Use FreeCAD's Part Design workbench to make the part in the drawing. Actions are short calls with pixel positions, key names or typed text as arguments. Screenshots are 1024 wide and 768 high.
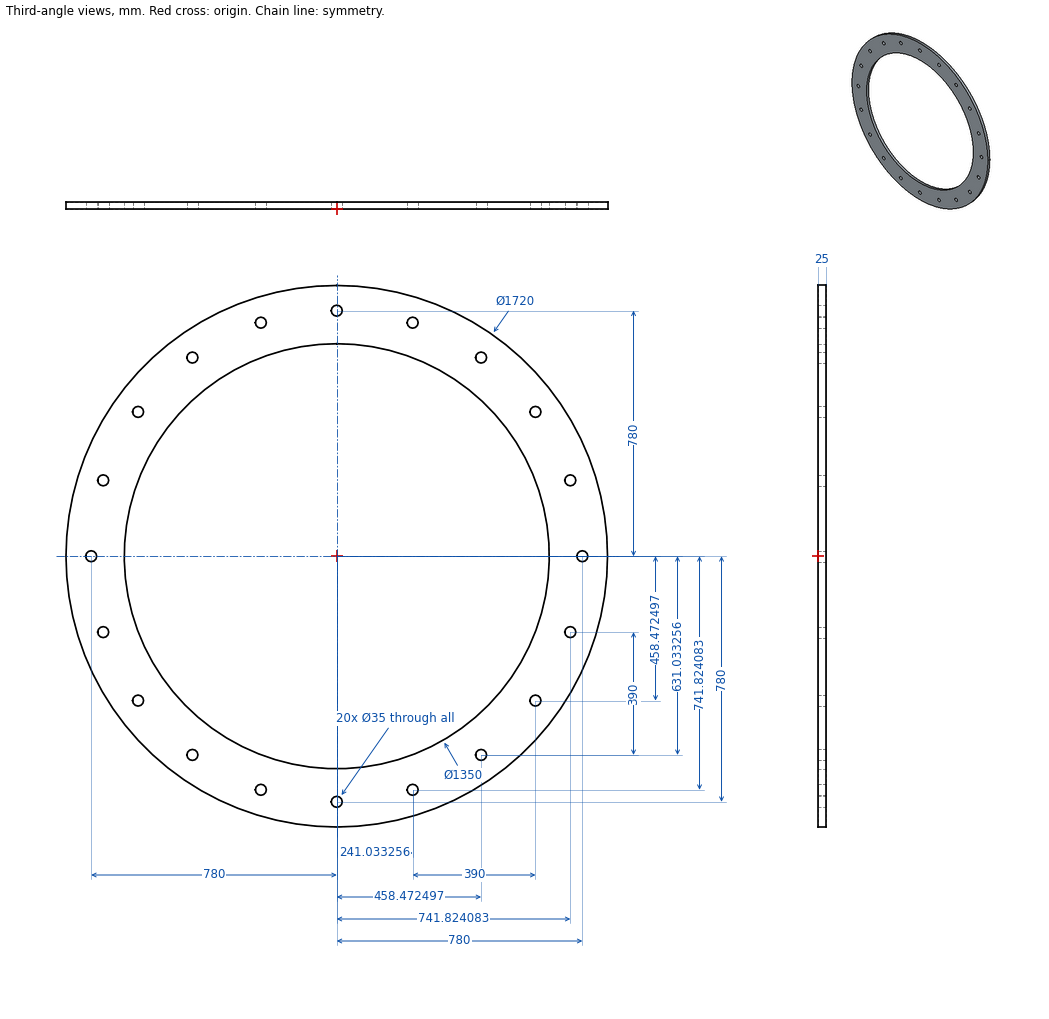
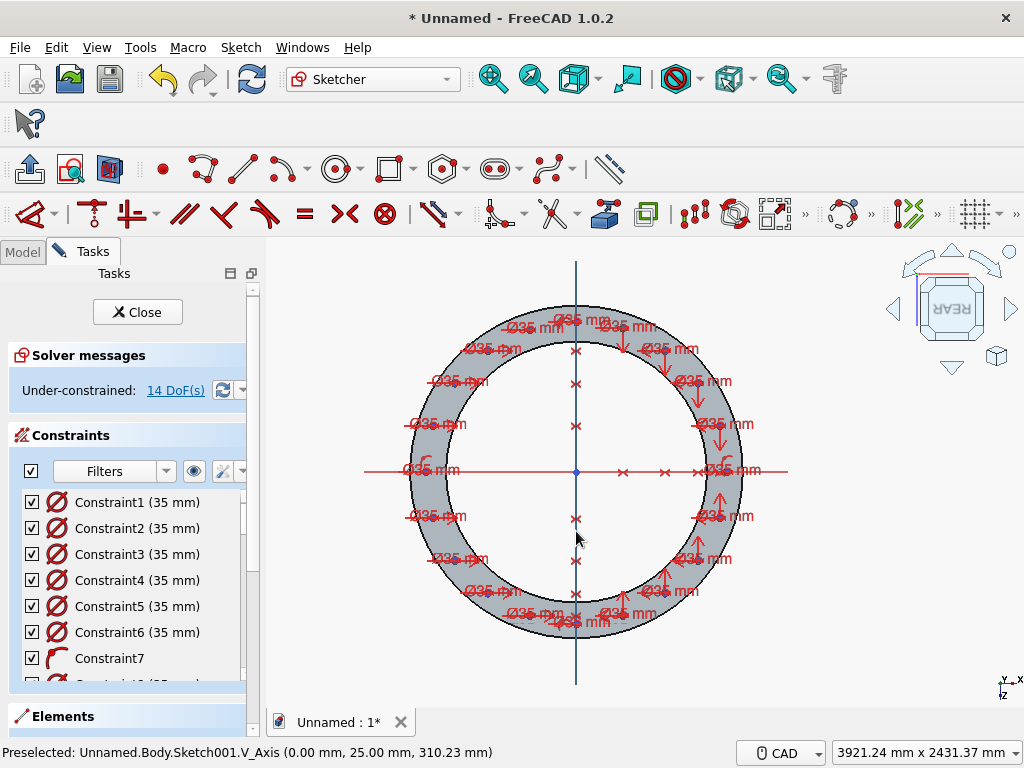
click(346, 214)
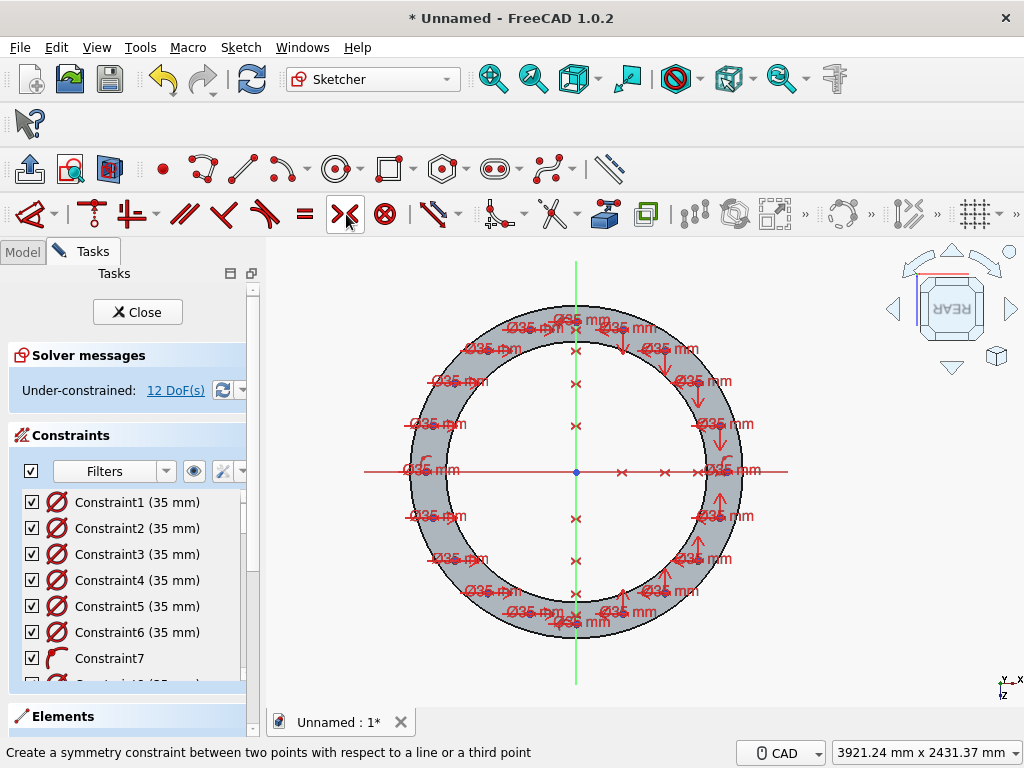
click(30, 214)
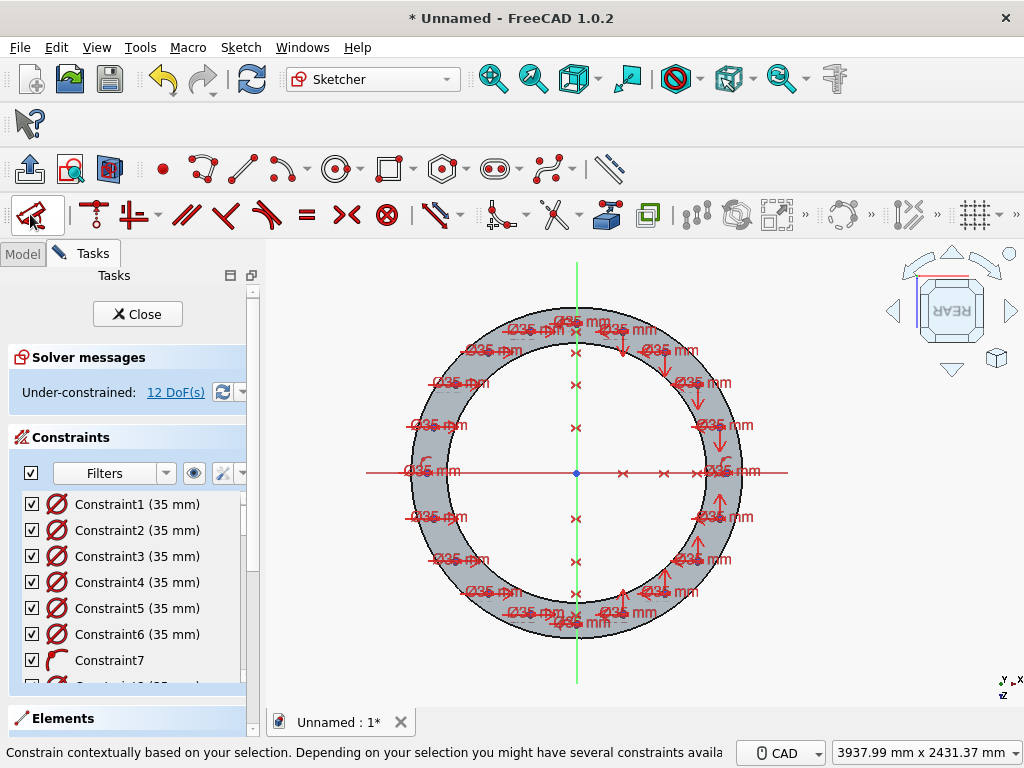
click(577, 324)
click(611, 398)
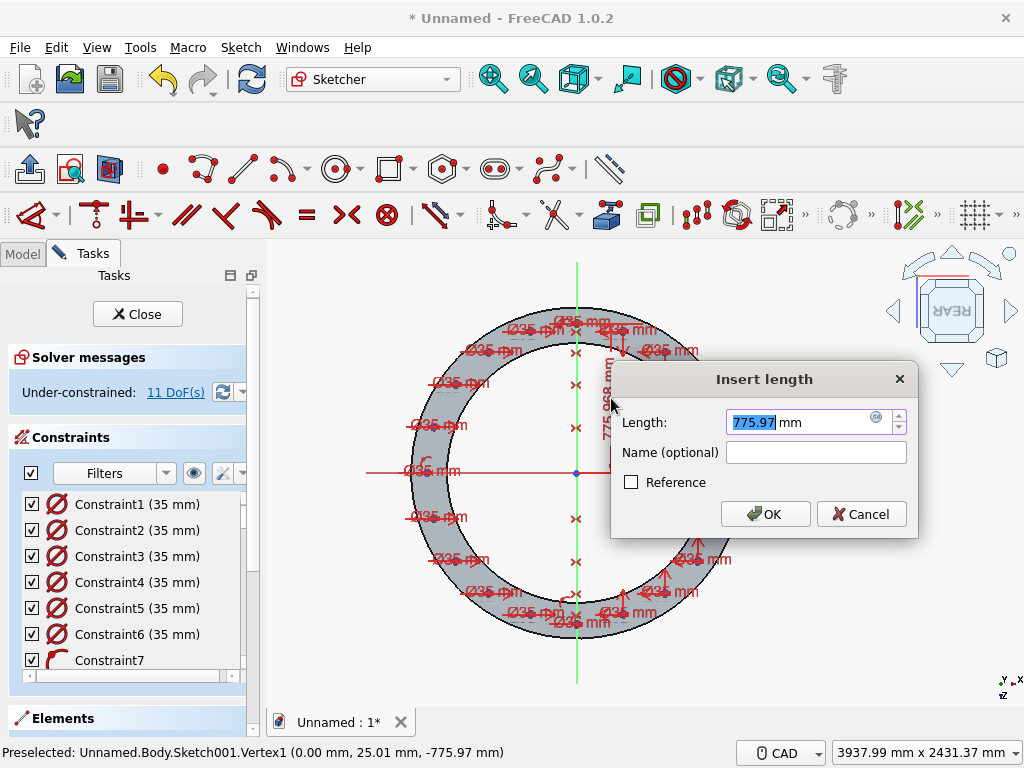
text(780)
key(Return)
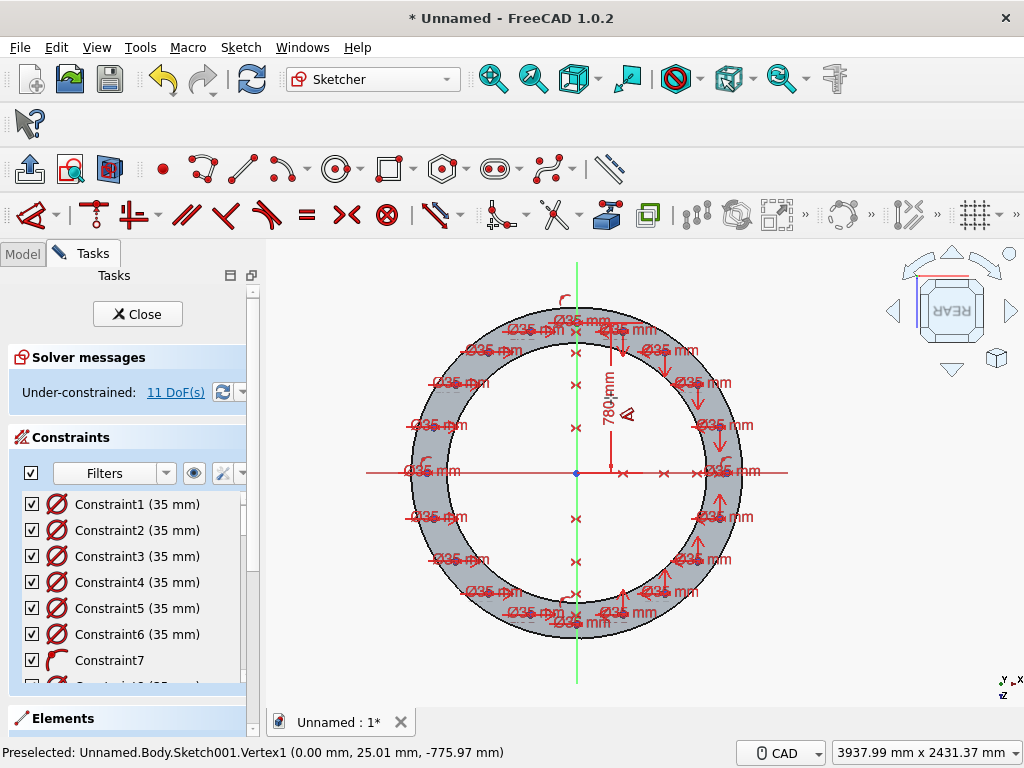
click(727, 473)
click(652, 507)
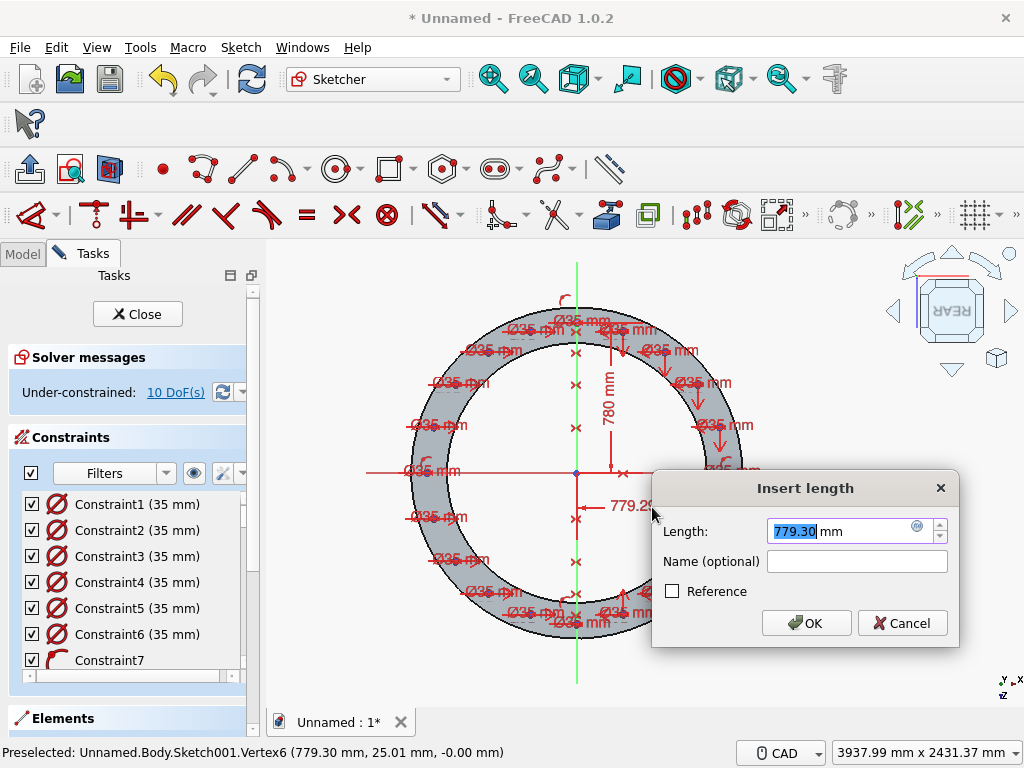
text(780)
key(Return)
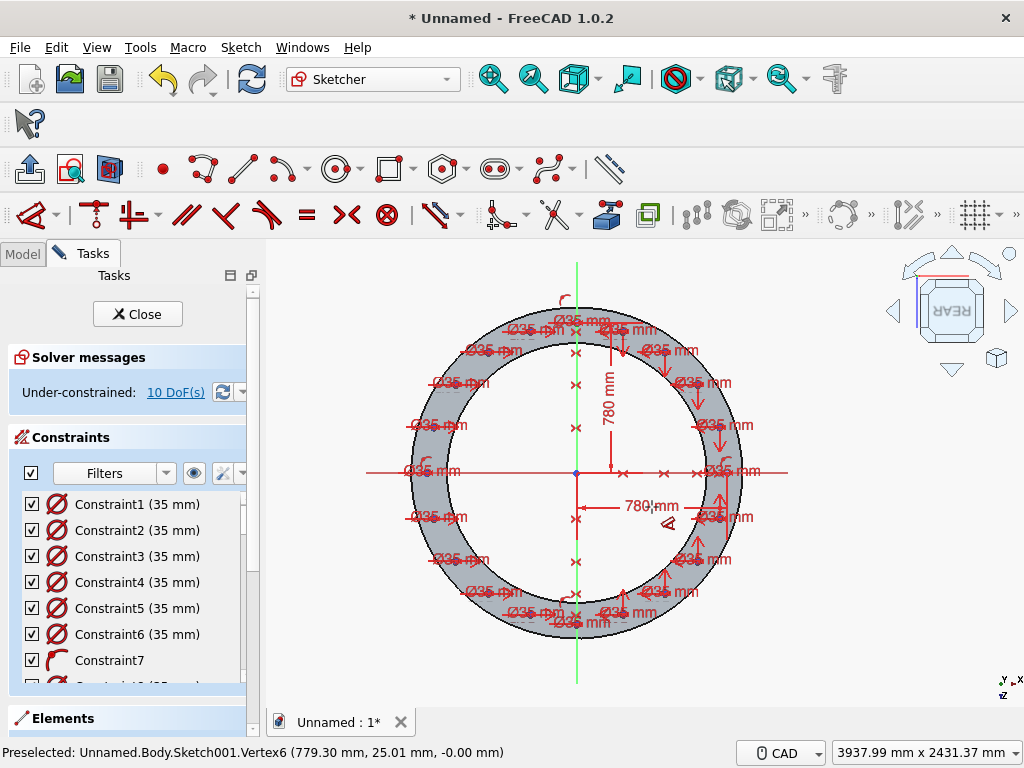
click(577, 624)
click(611, 549)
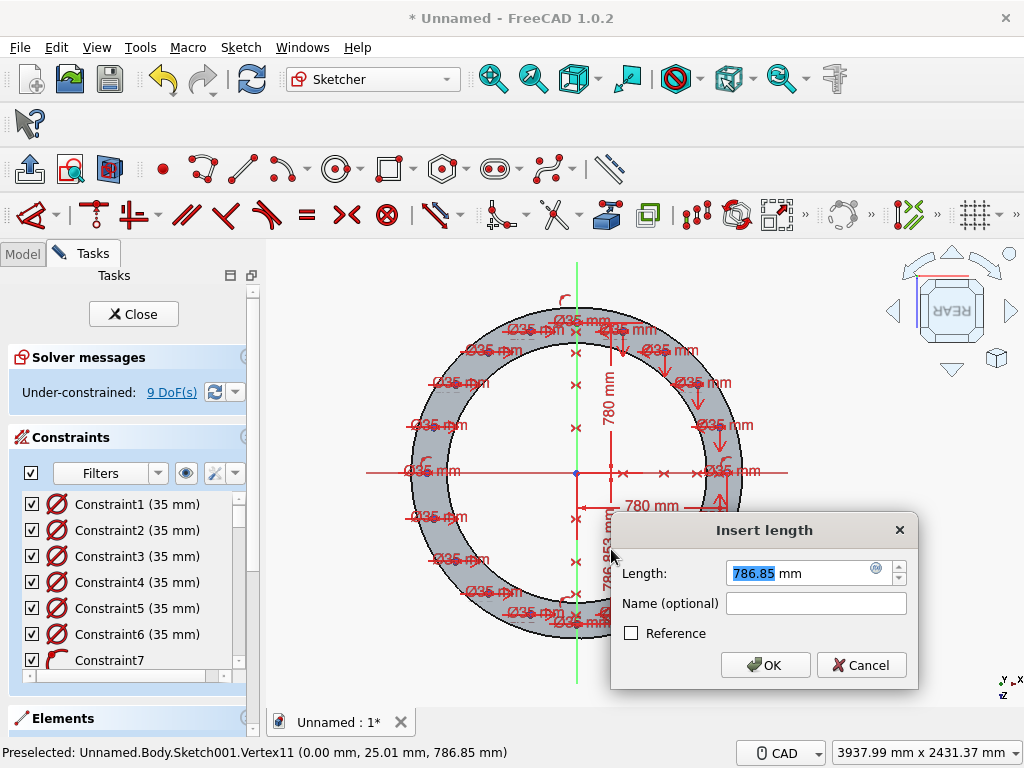
text(780)
key(Return)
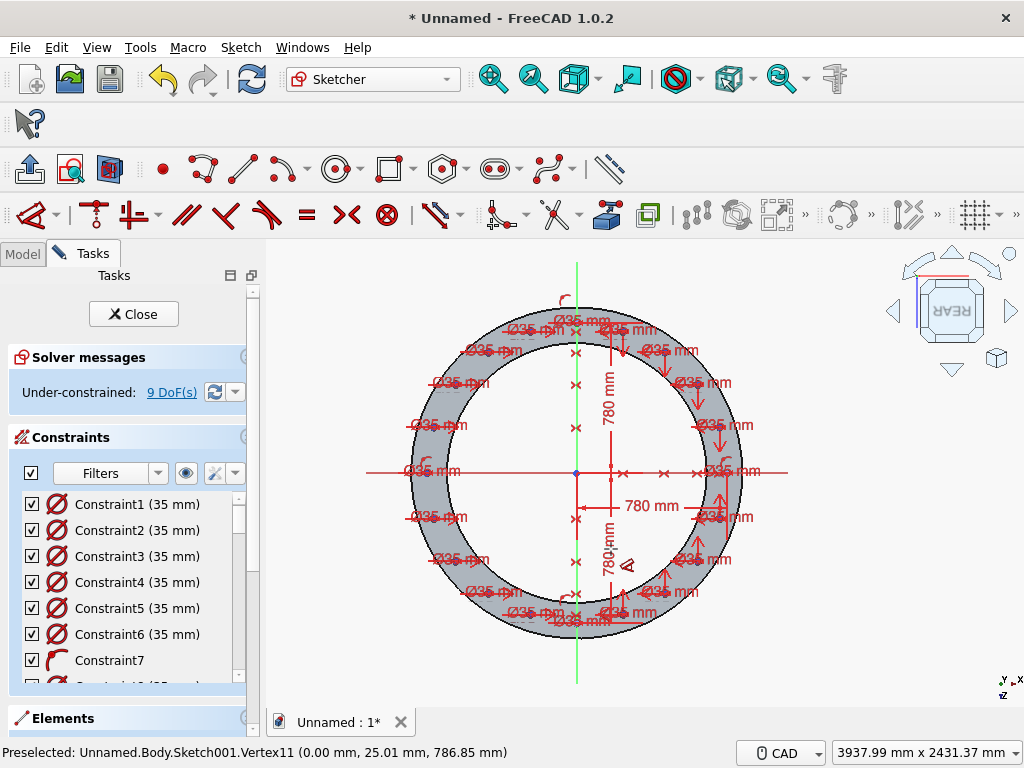
click(427, 473)
click(502, 507)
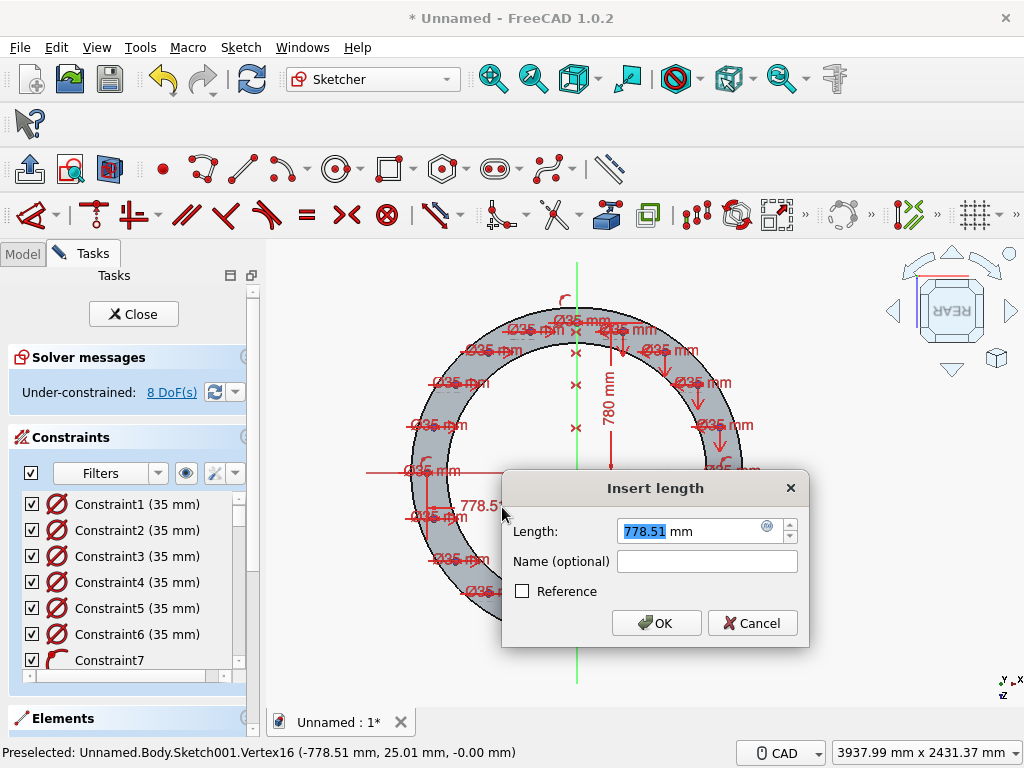
text(780)
key(Return)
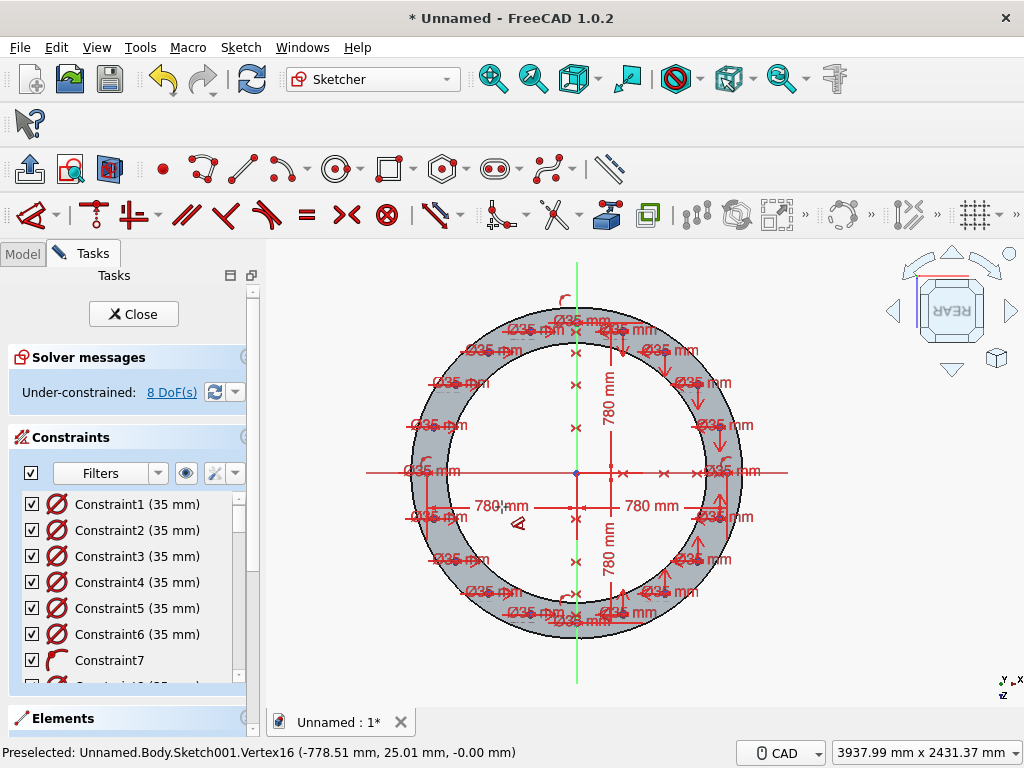
click(623, 332)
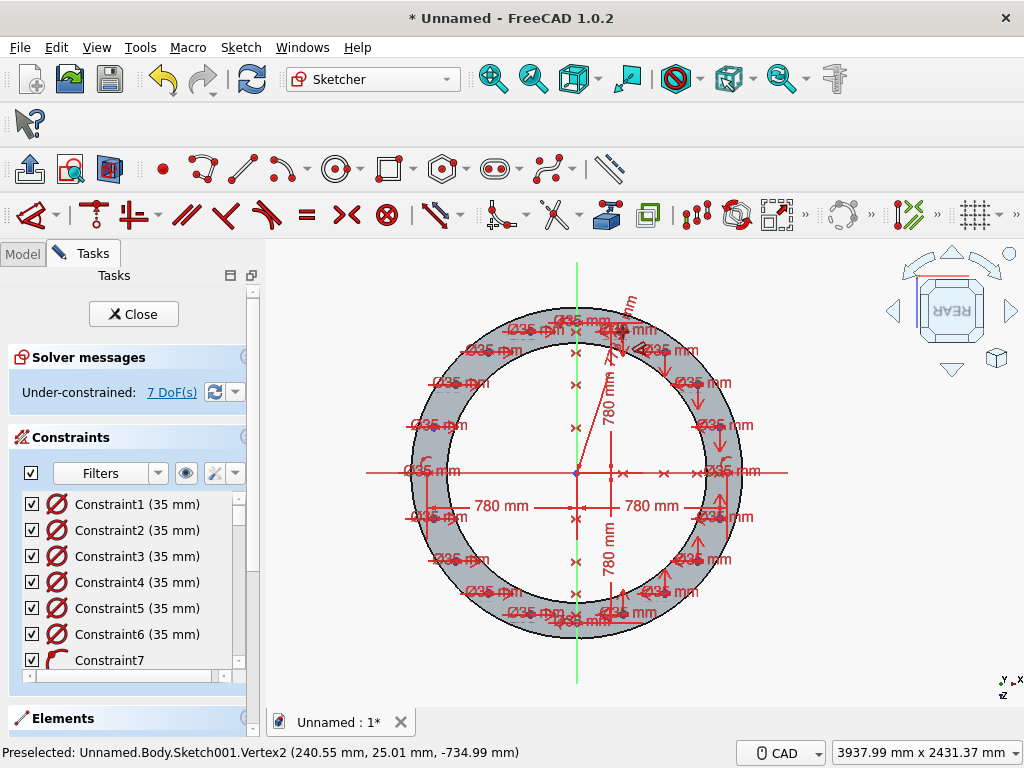
click(698, 385)
click(660, 298)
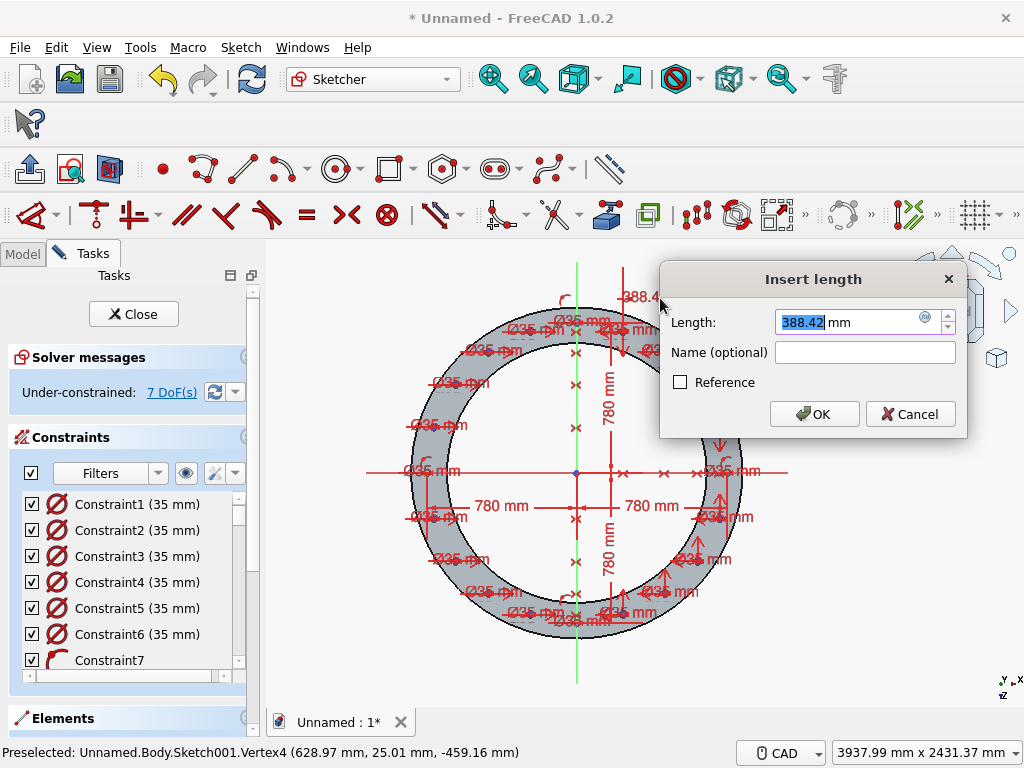
text(390)
key(Return)